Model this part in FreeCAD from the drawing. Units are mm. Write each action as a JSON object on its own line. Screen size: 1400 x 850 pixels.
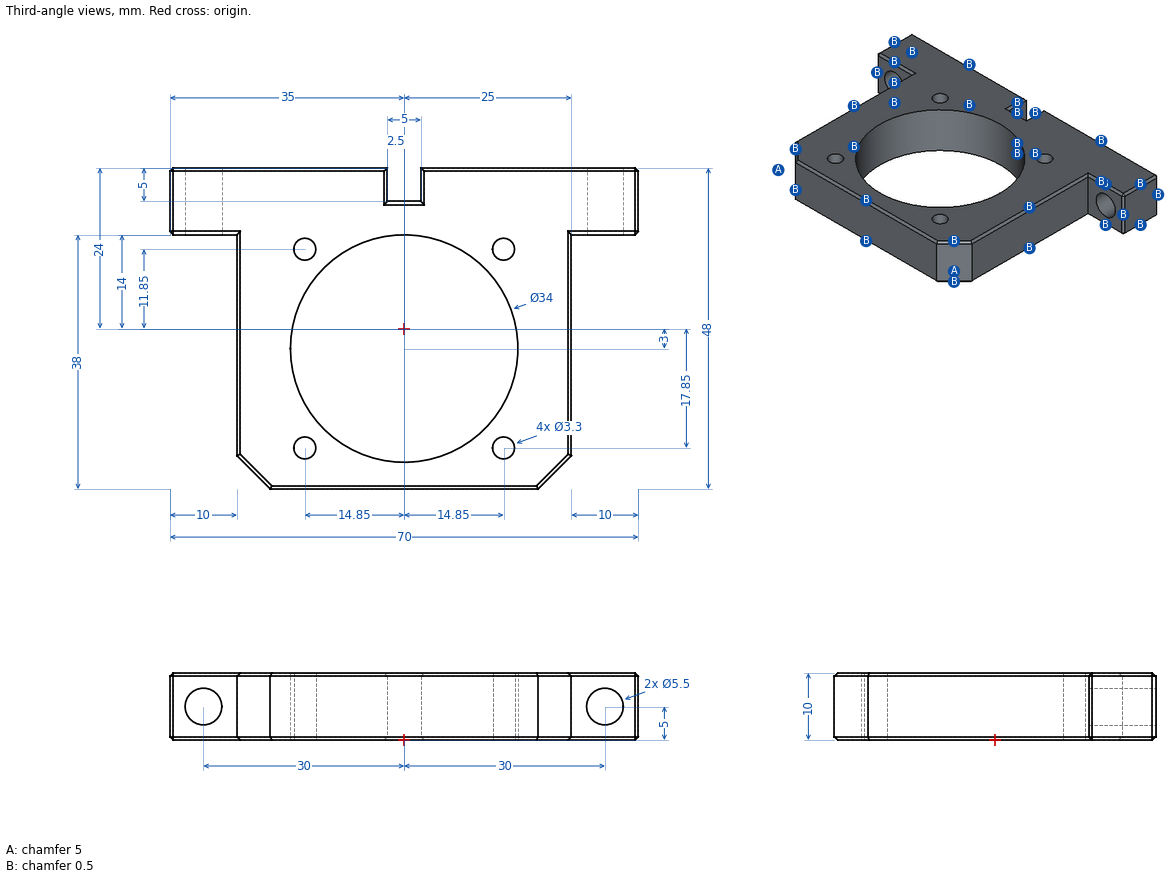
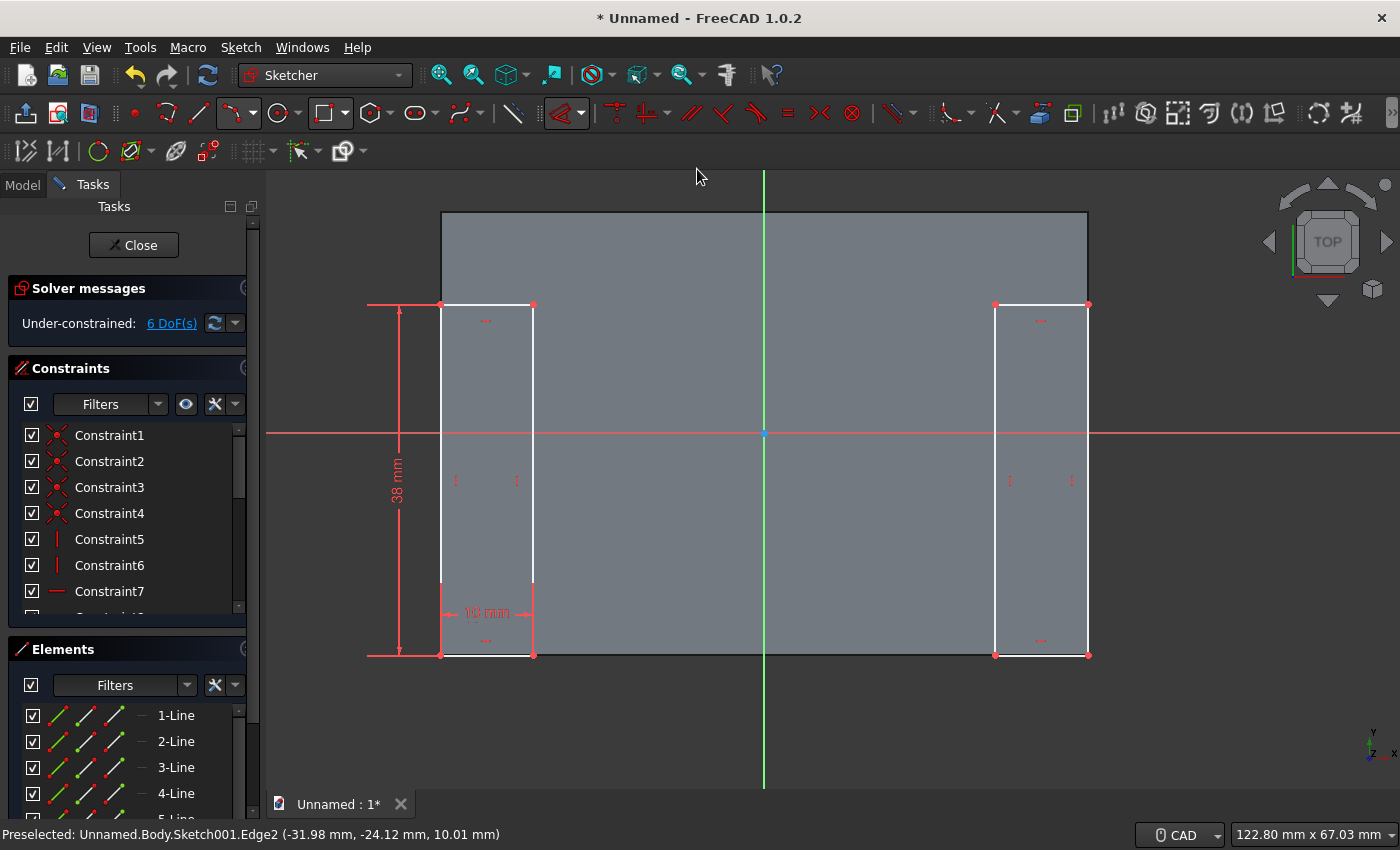
{"action": "left_click", "coordinate": [995, 410]}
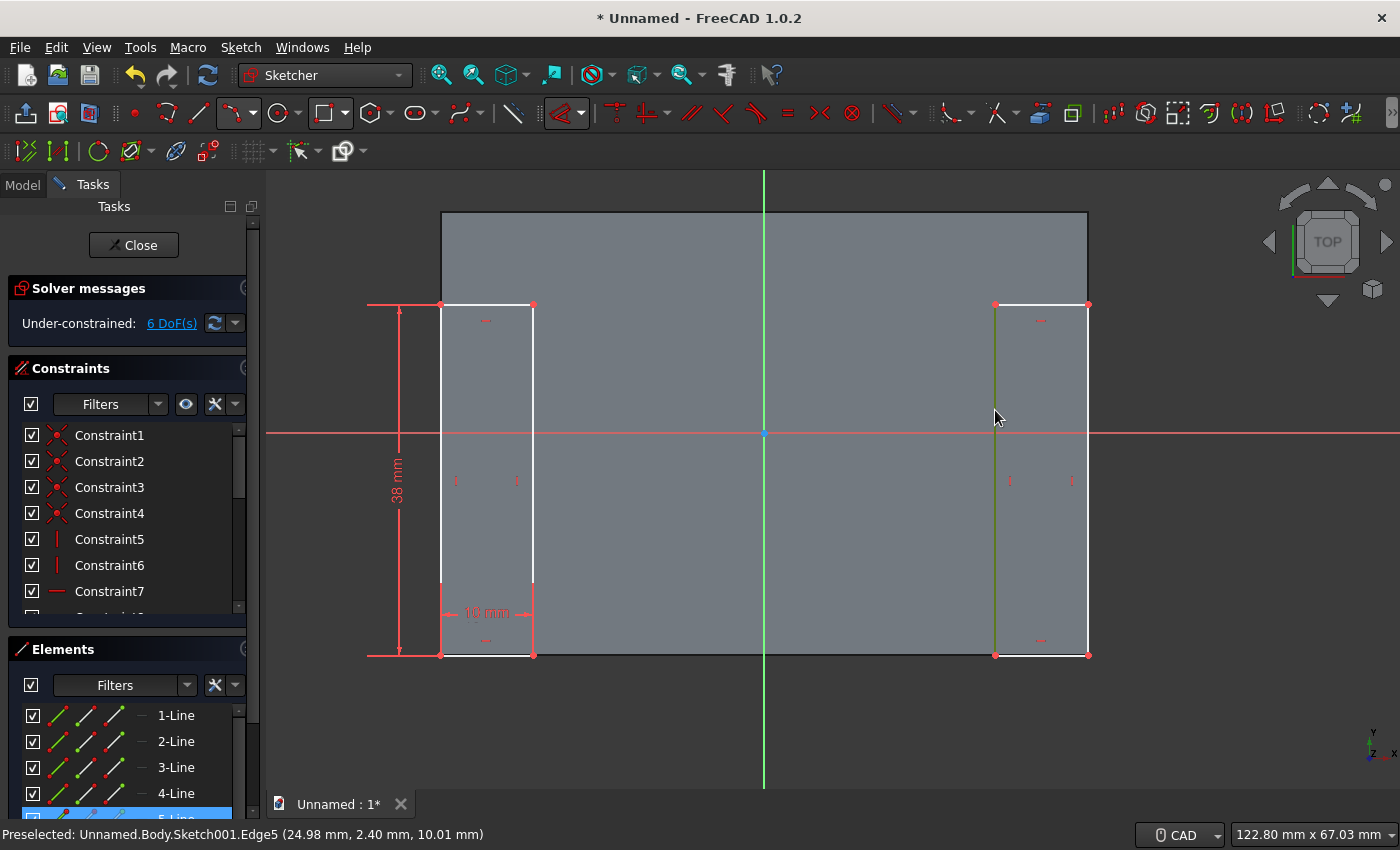
{"action": "left_click", "coordinate": [584, 114]}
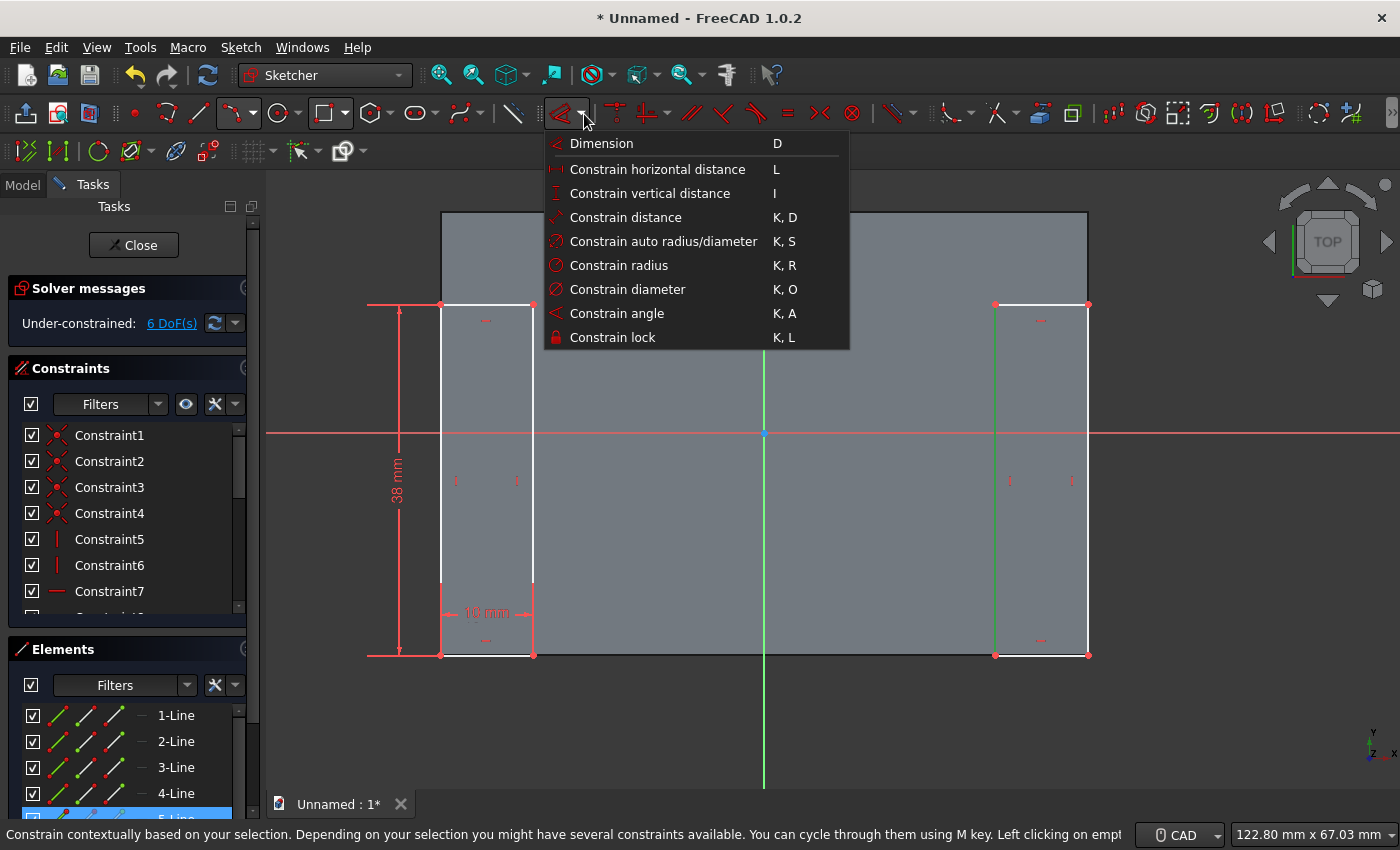
{"action": "left_click", "coordinate": [697, 193]}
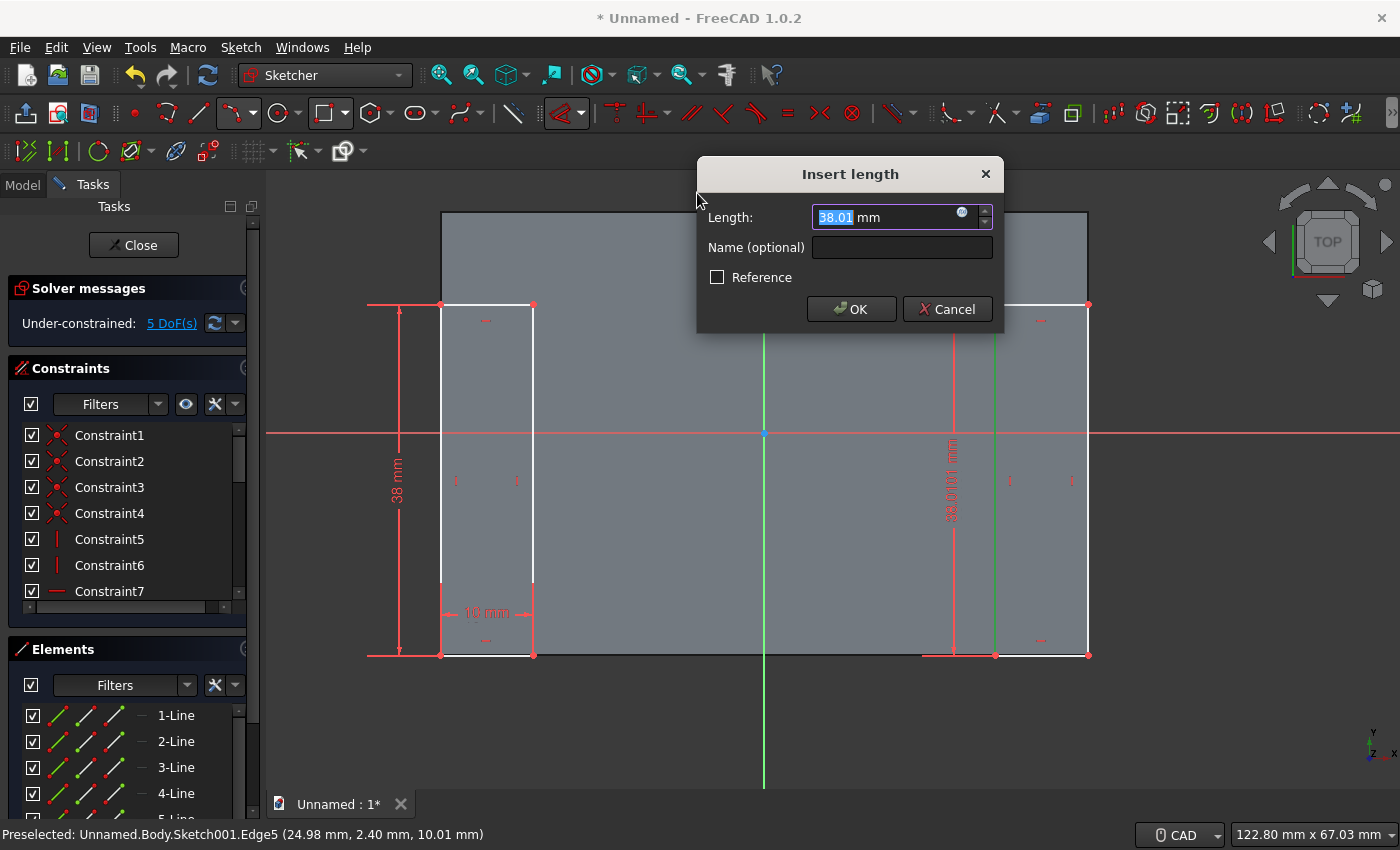
{"action": "type", "text": "38"}
{"action": "key", "text": "Return"}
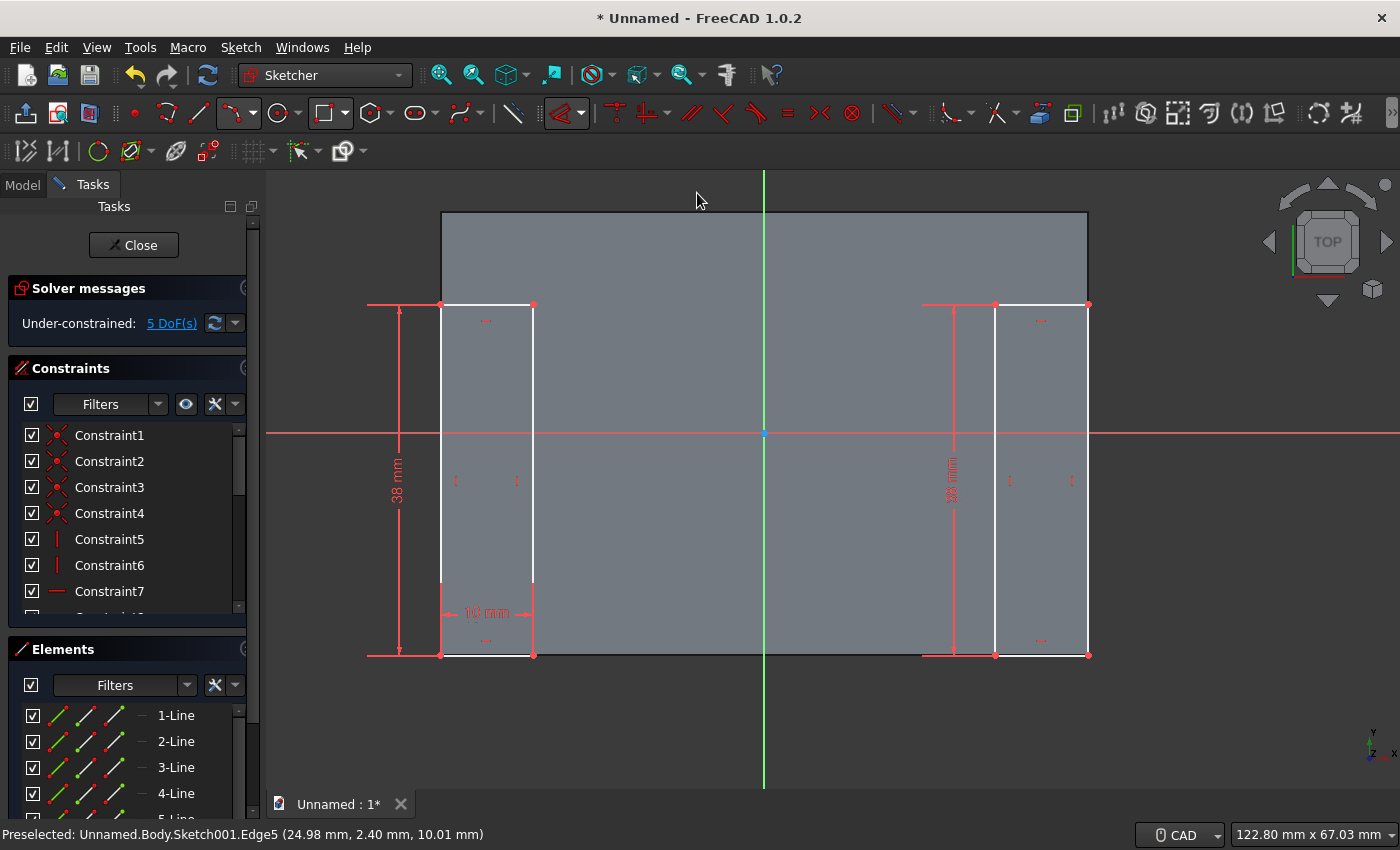
{"action": "left_click", "coordinate": [1023, 656]}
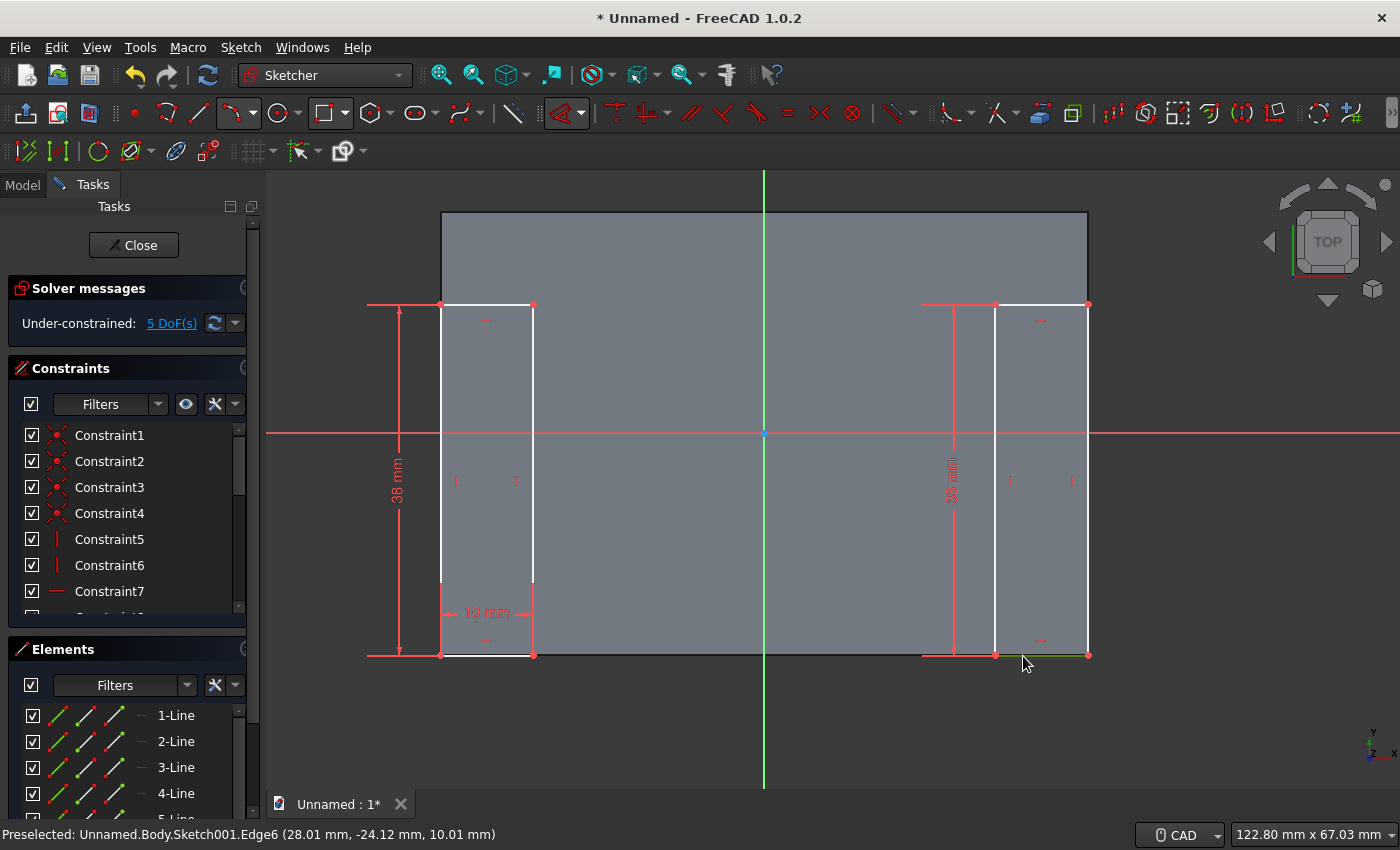
{"action": "left_click", "coordinate": [584, 114]}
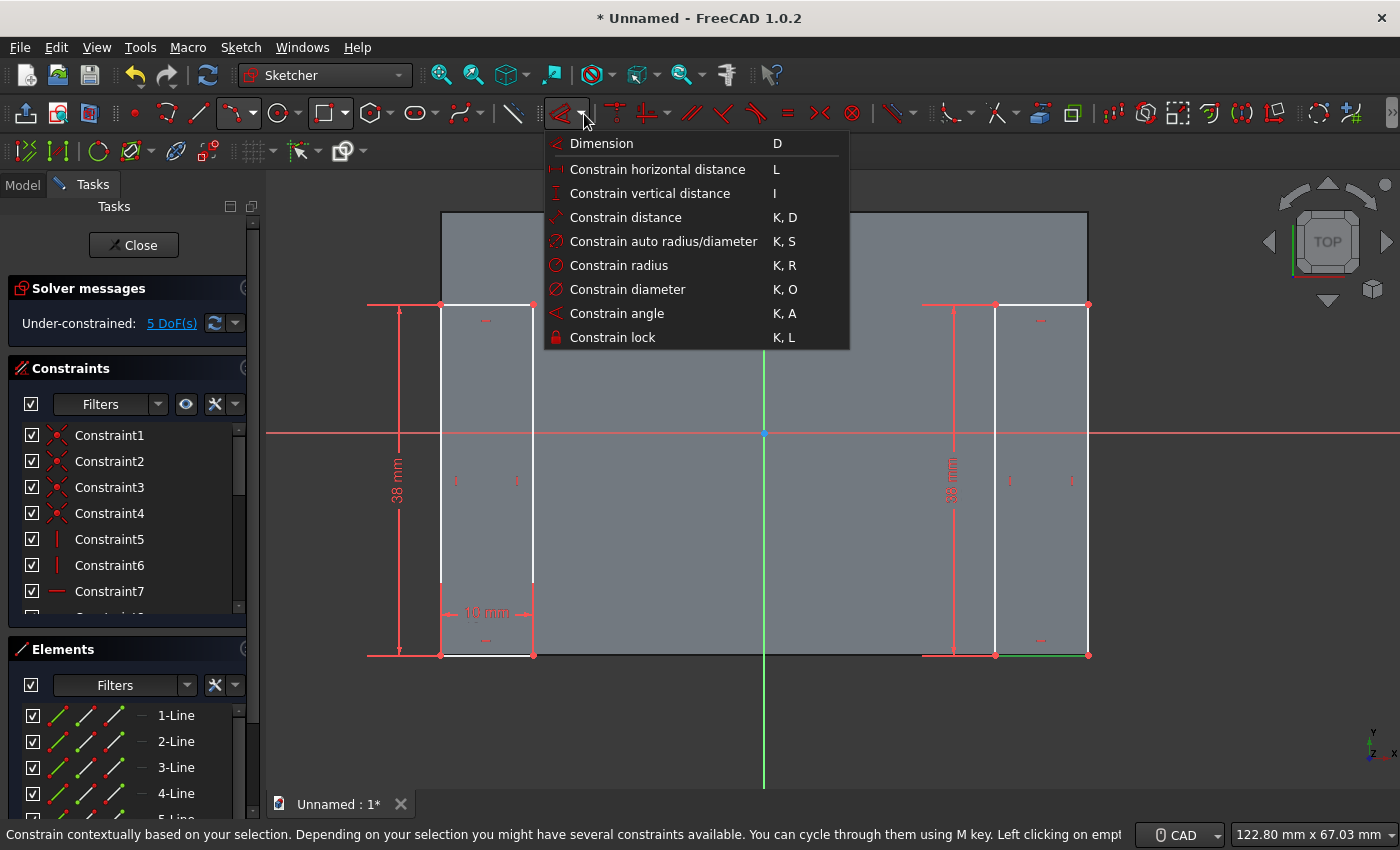
{"action": "left_click", "coordinate": [697, 169]}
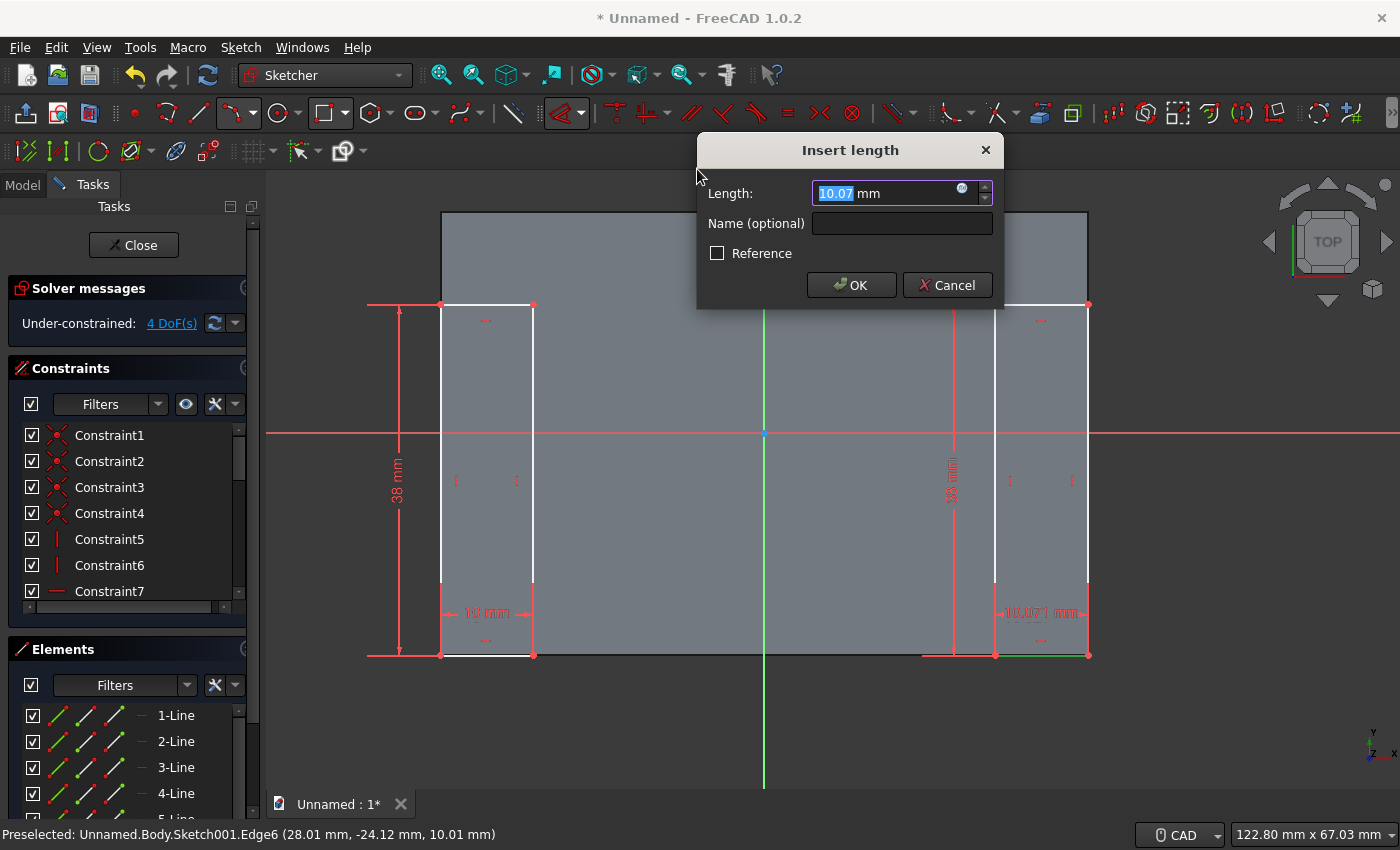
{"action": "type", "text": "10"}
{"action": "key", "text": "Return"}